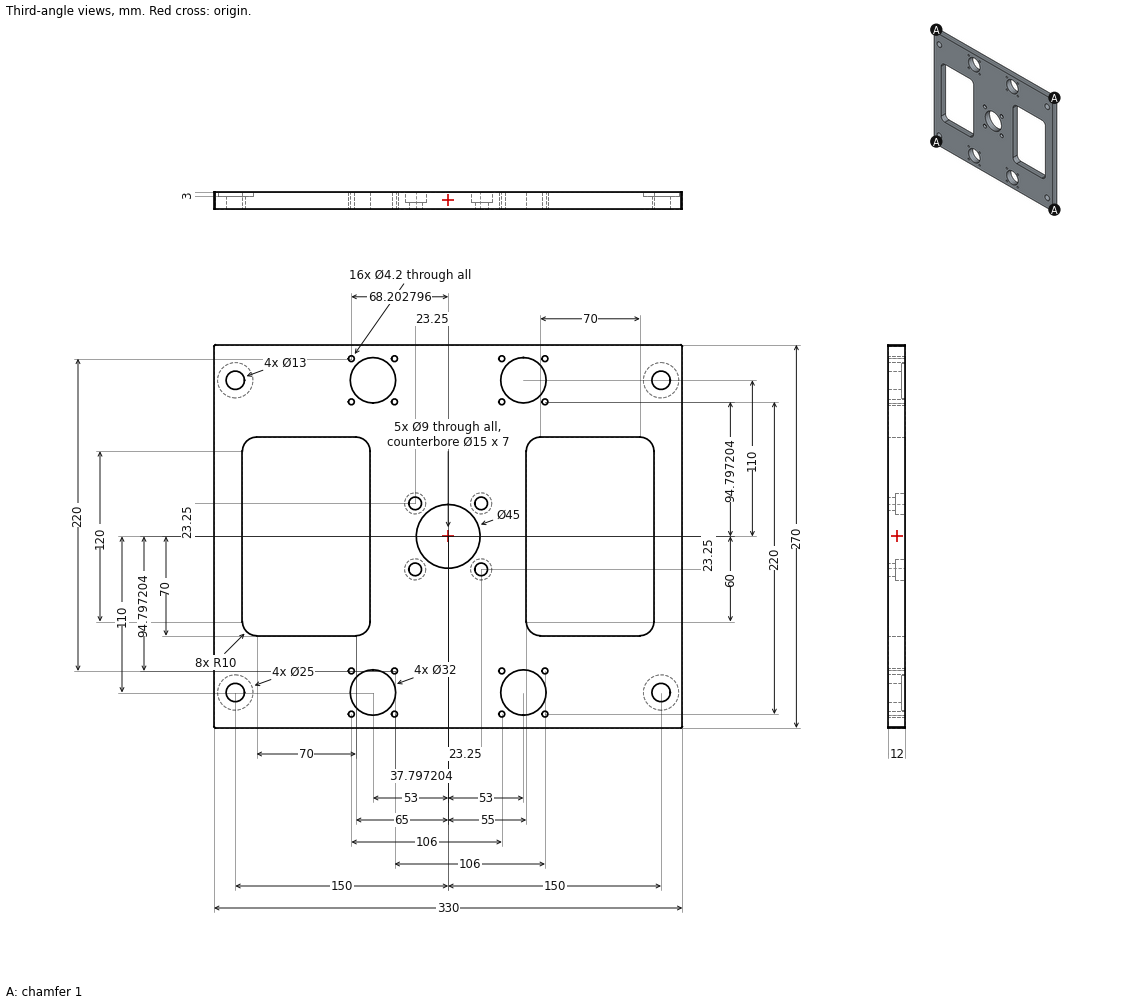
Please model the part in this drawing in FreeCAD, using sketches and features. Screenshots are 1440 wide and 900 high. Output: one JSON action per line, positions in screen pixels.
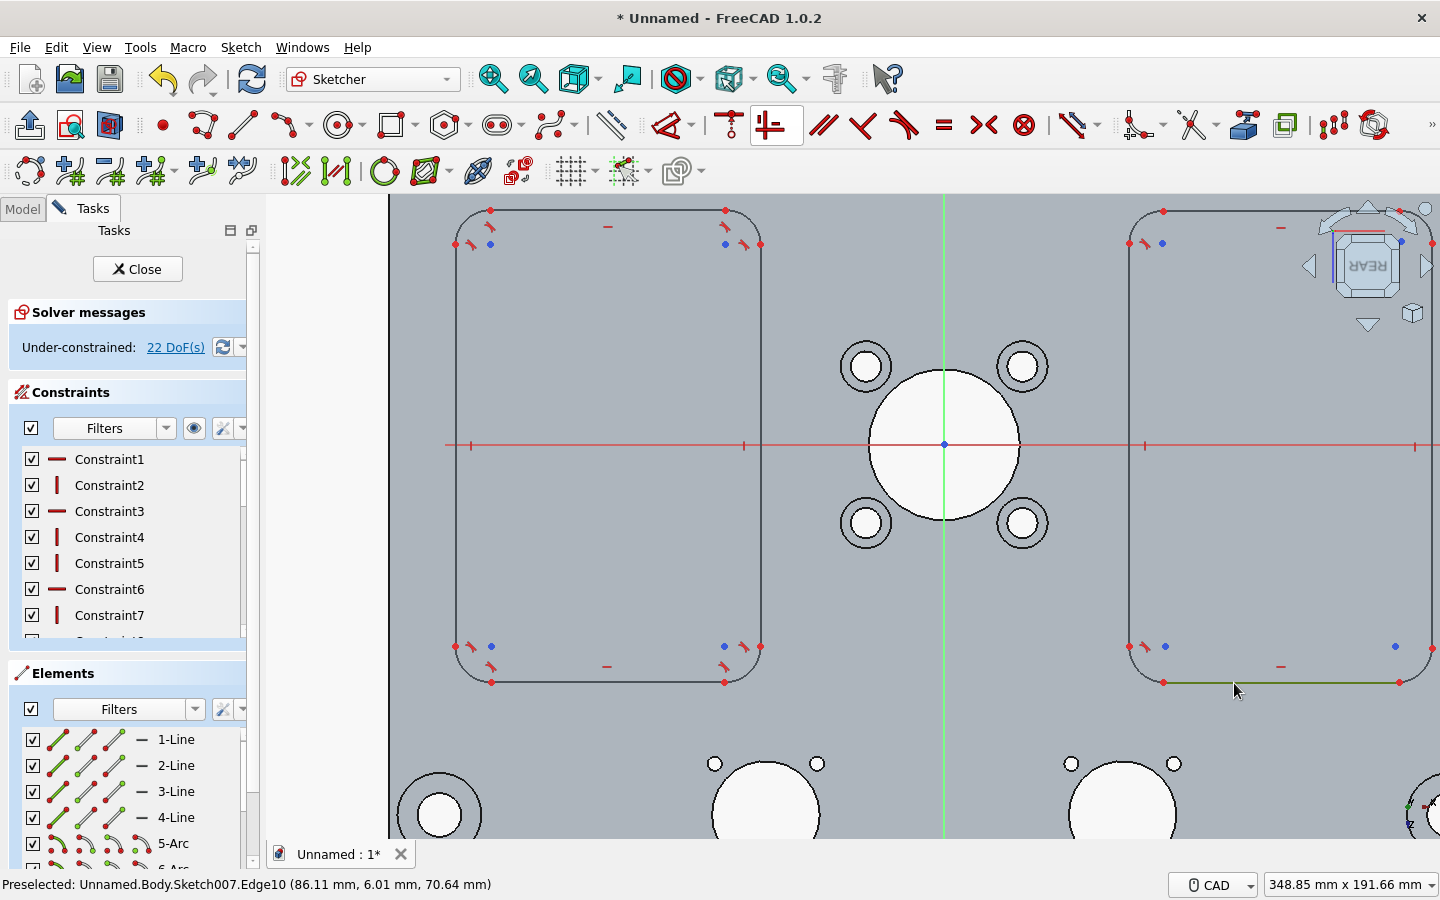
{"action": "left_click", "coordinate": [1133, 662]}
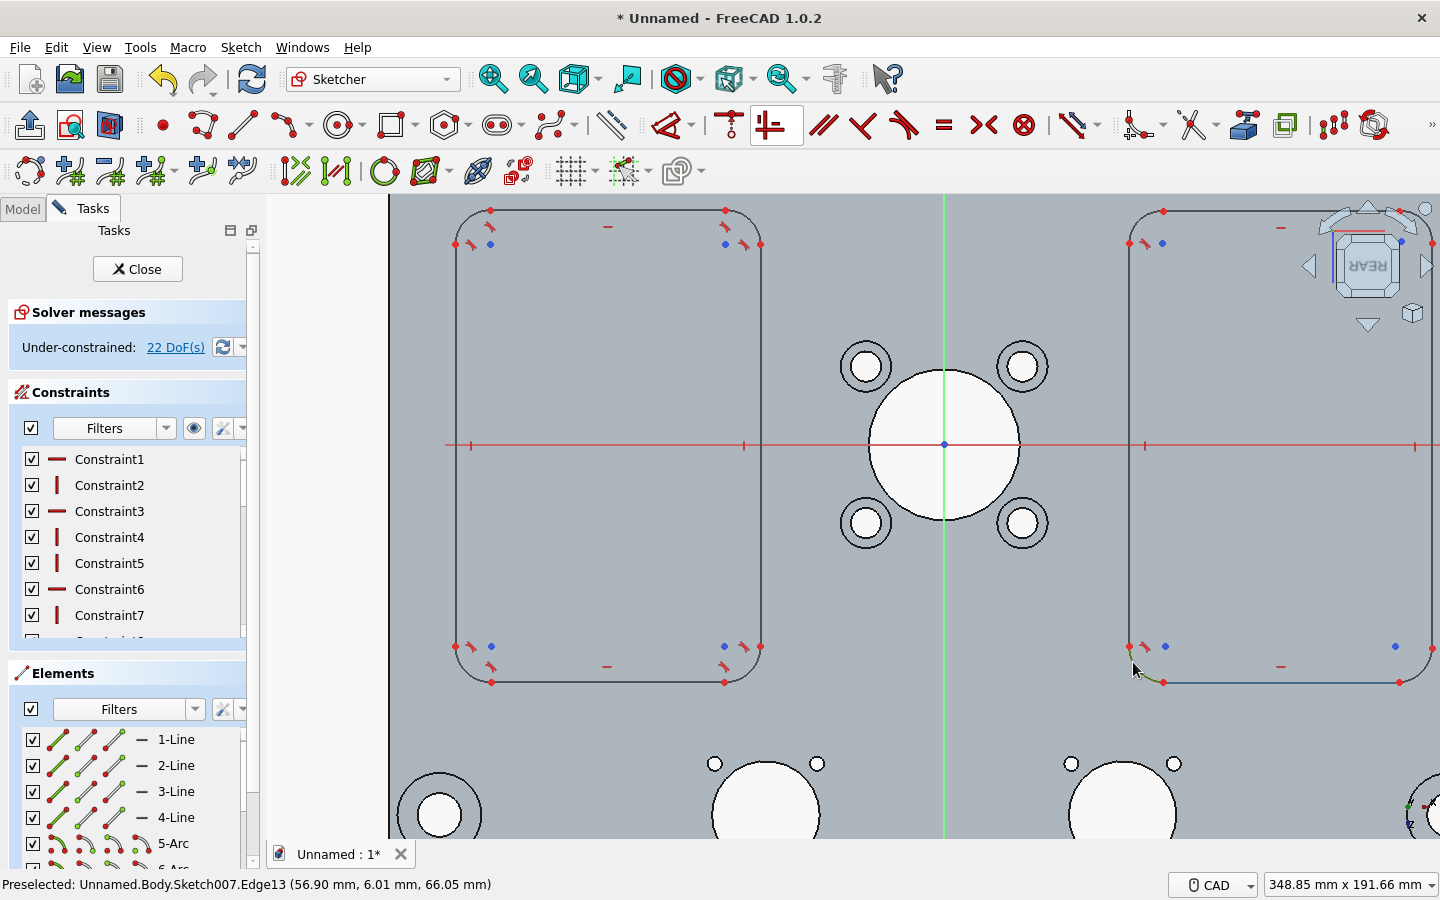
{"action": "left_click", "coordinate": [904, 126]}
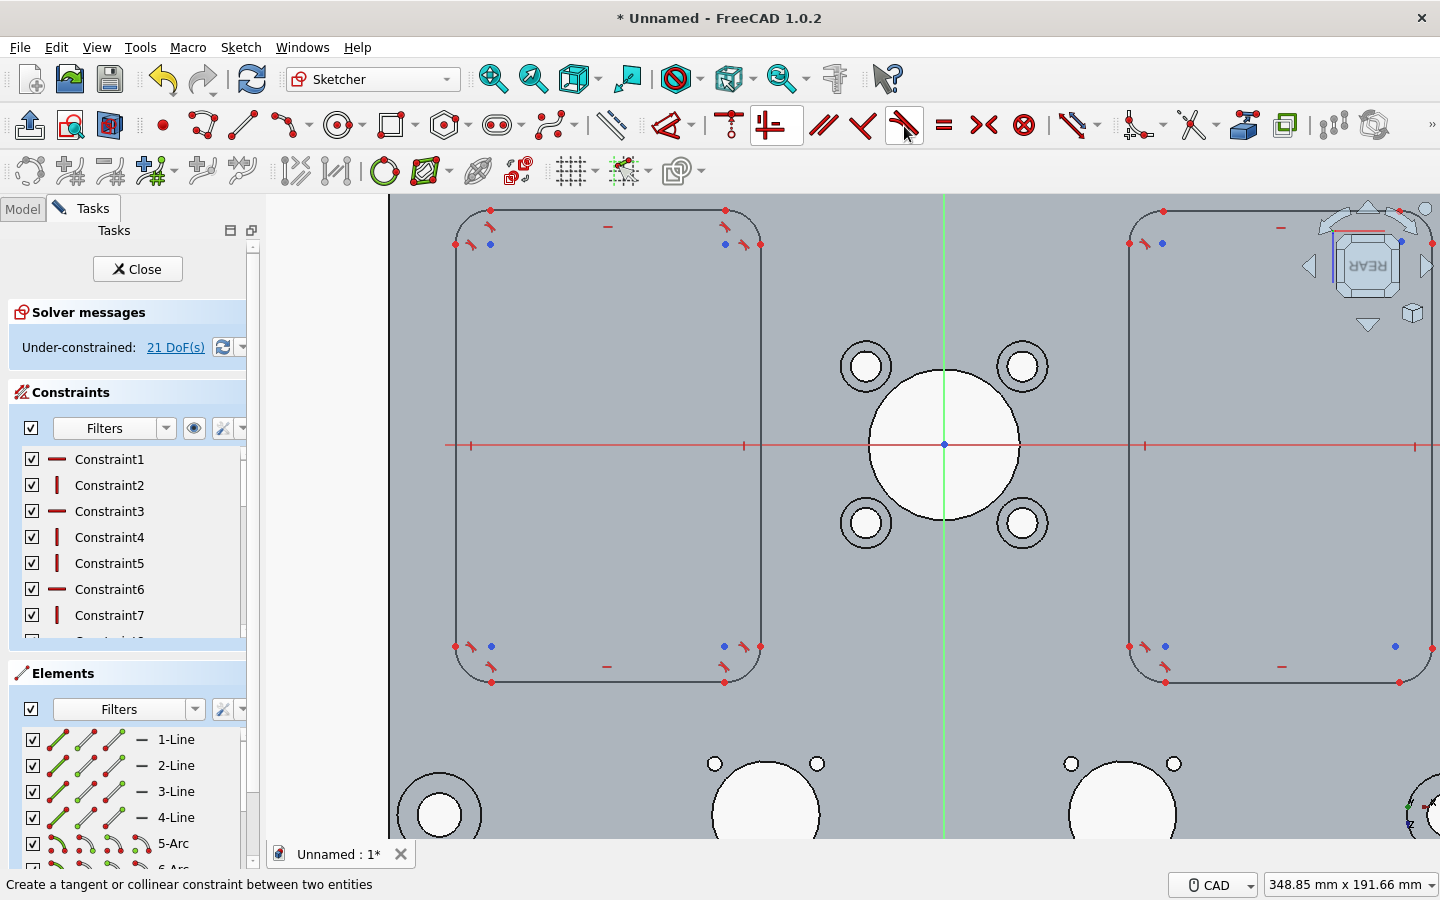
{"action": "left_click", "coordinate": [1236, 683]}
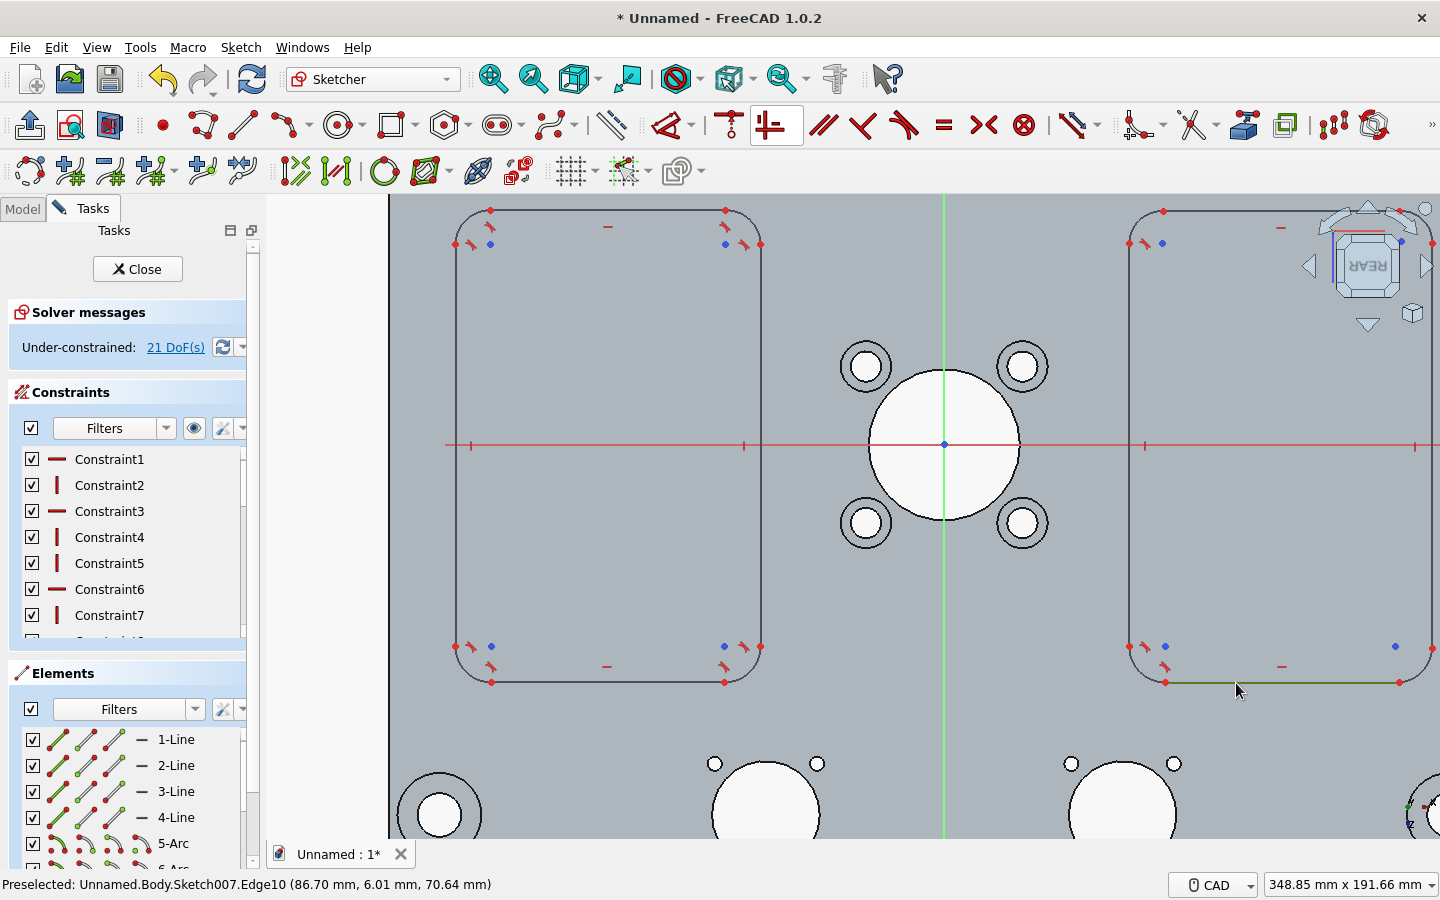
{"action": "scroll", "coordinate": [460, 662], "scroll_direction": "down", "scroll_amount": 2}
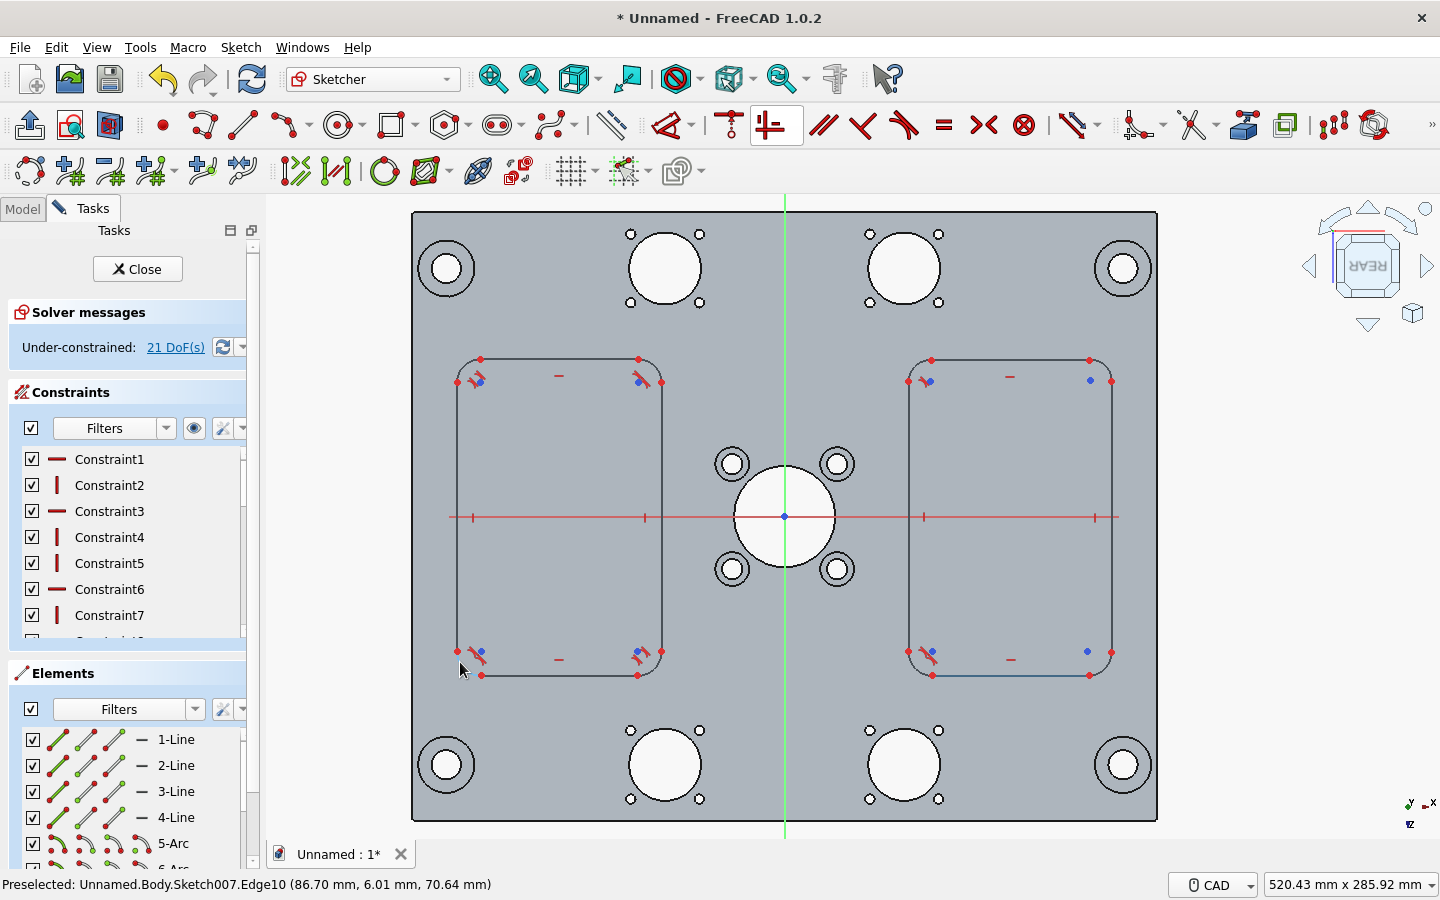
{"action": "scroll", "coordinate": [1100, 673], "scroll_direction": "up", "scroll_amount": 2}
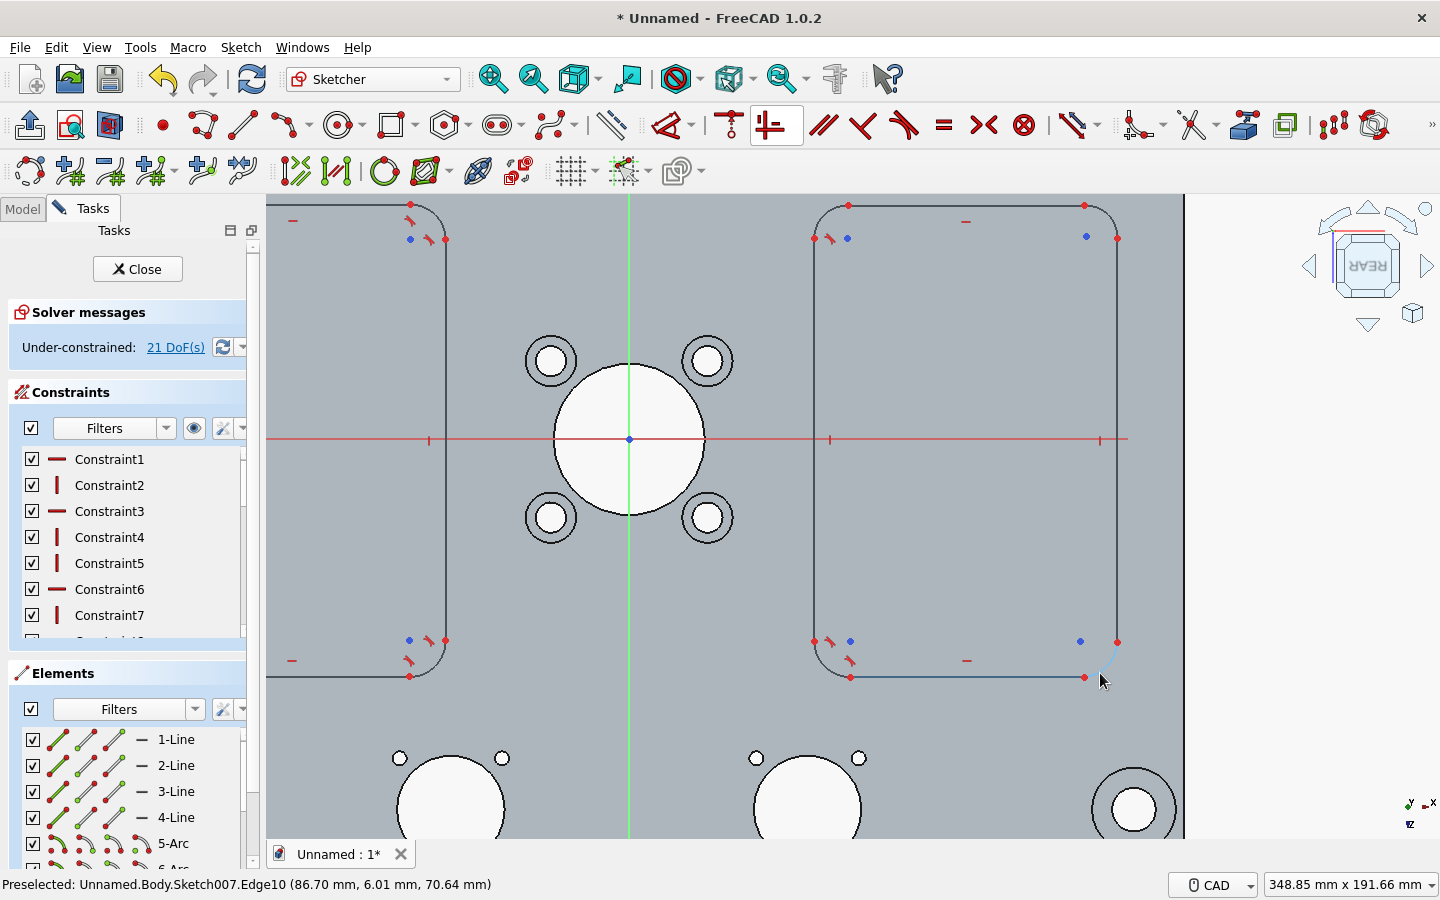
{"action": "left_click", "coordinate": [1099, 672]}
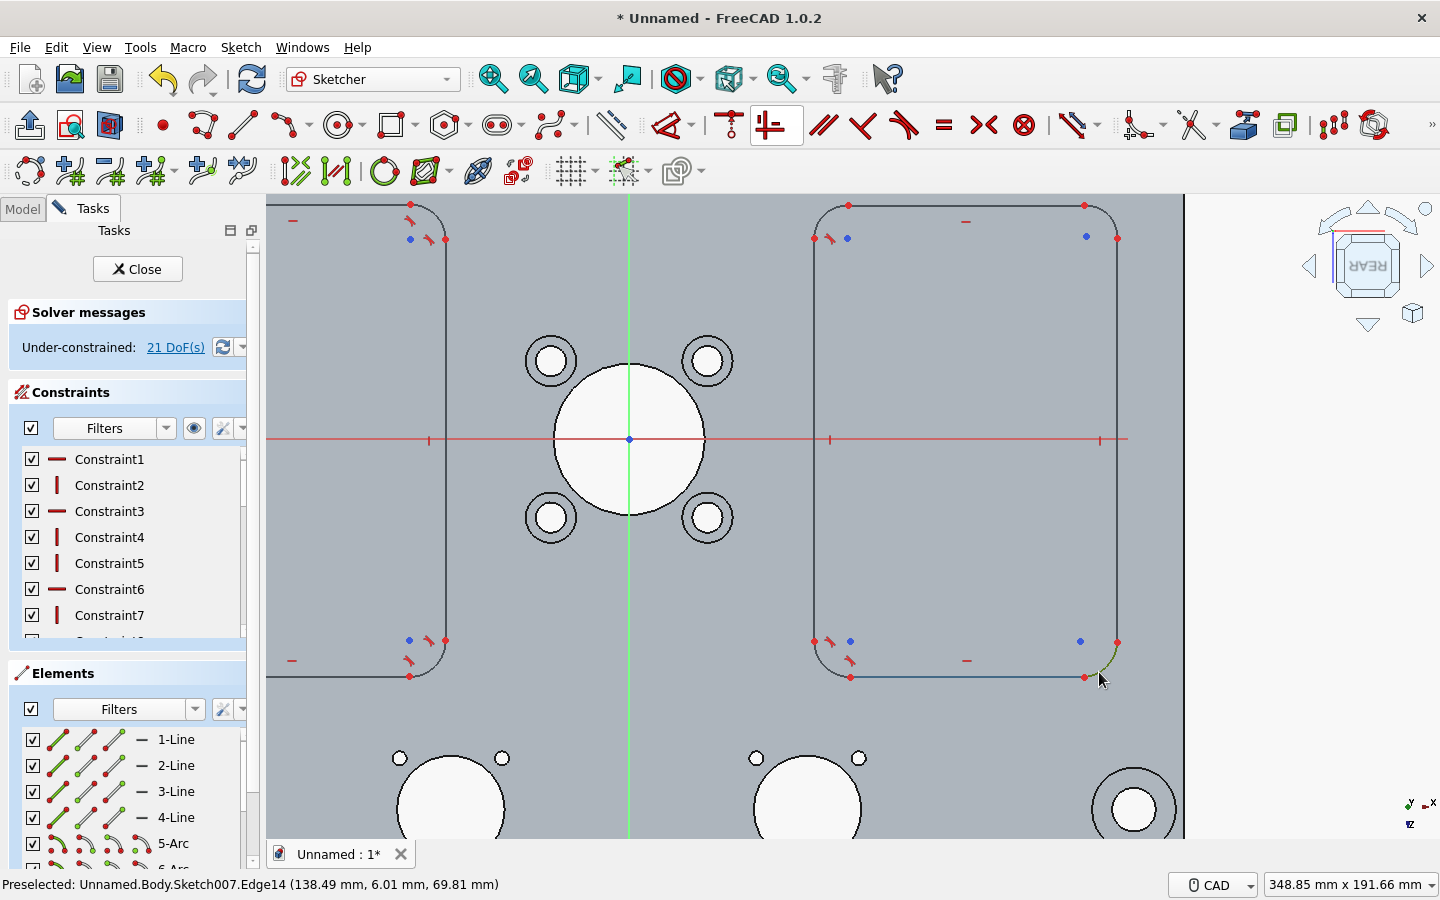
{"action": "left_click", "coordinate": [904, 126]}